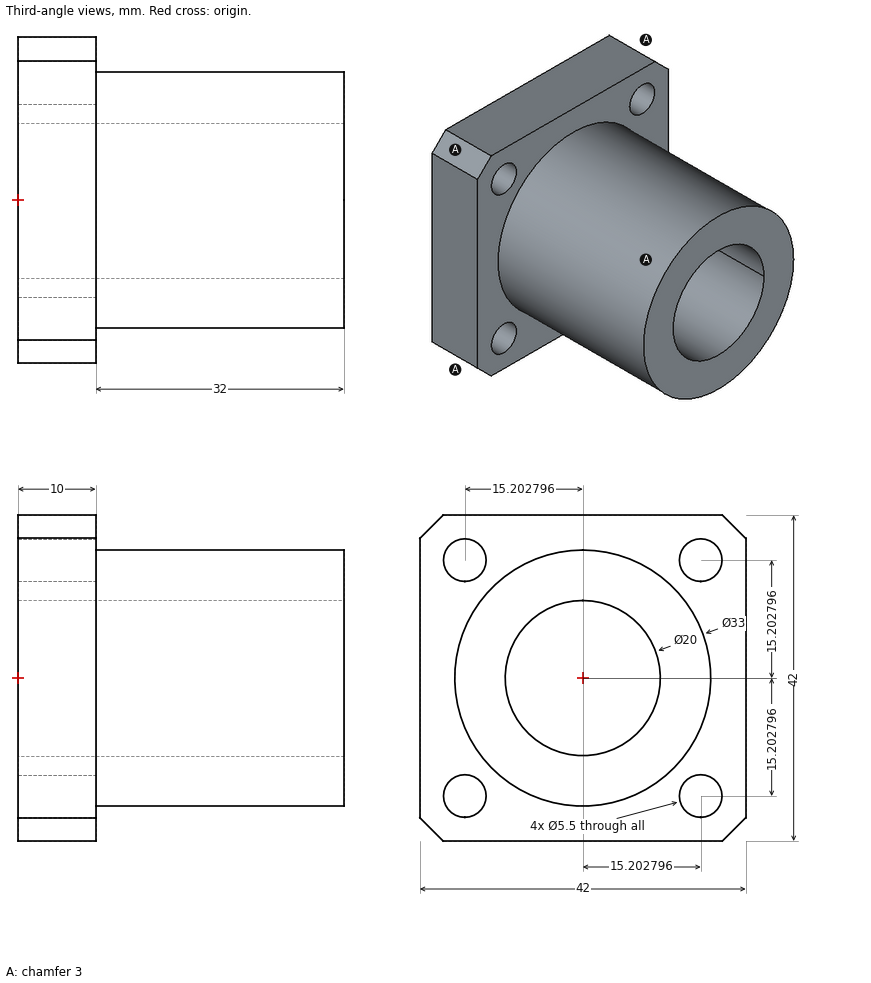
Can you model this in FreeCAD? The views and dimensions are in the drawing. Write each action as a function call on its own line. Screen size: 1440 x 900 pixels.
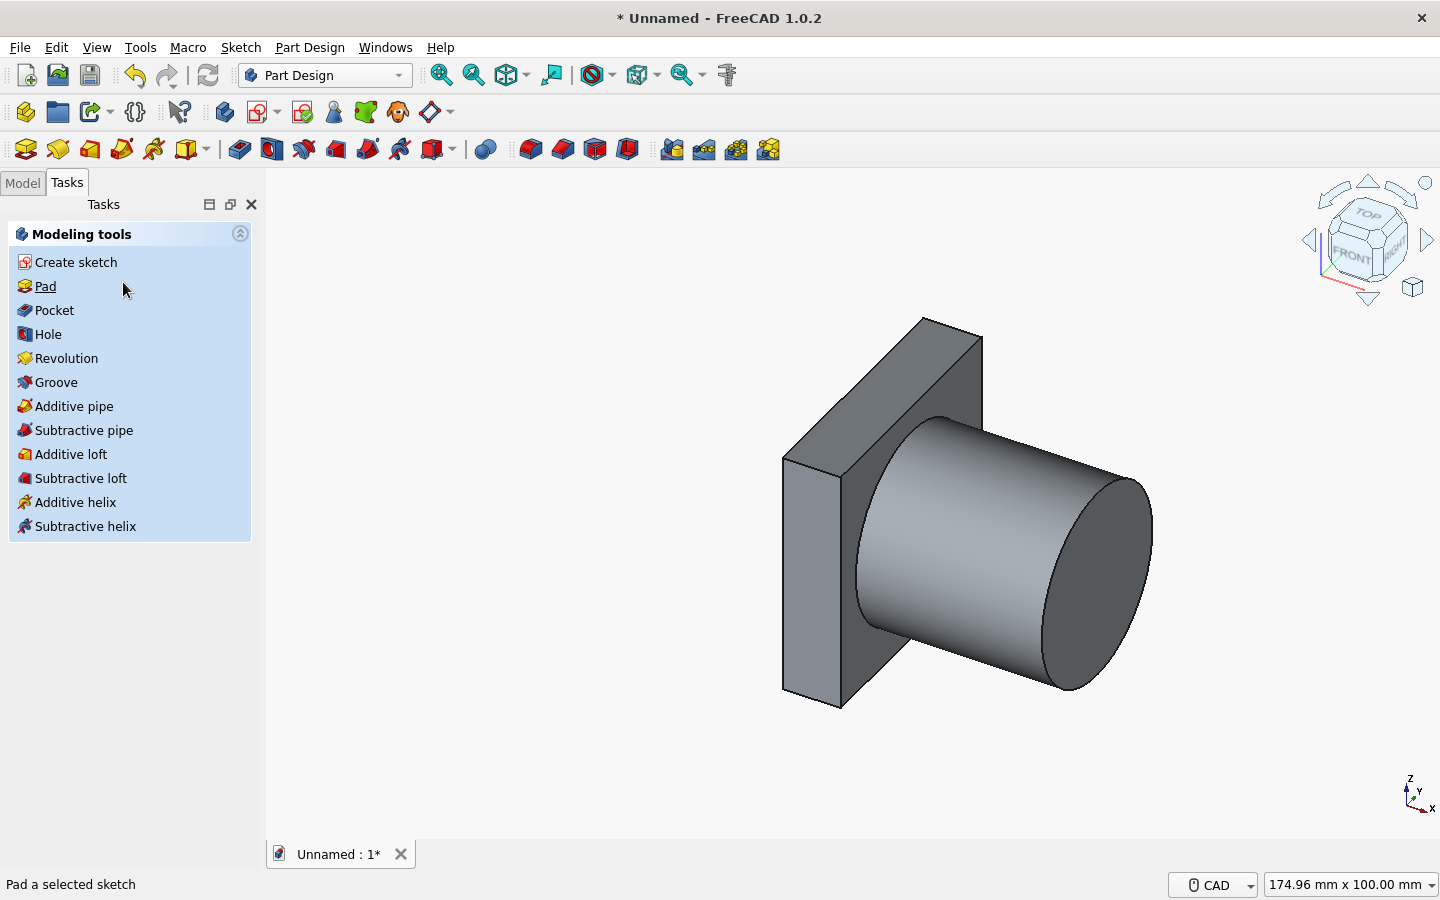
click(272, 150)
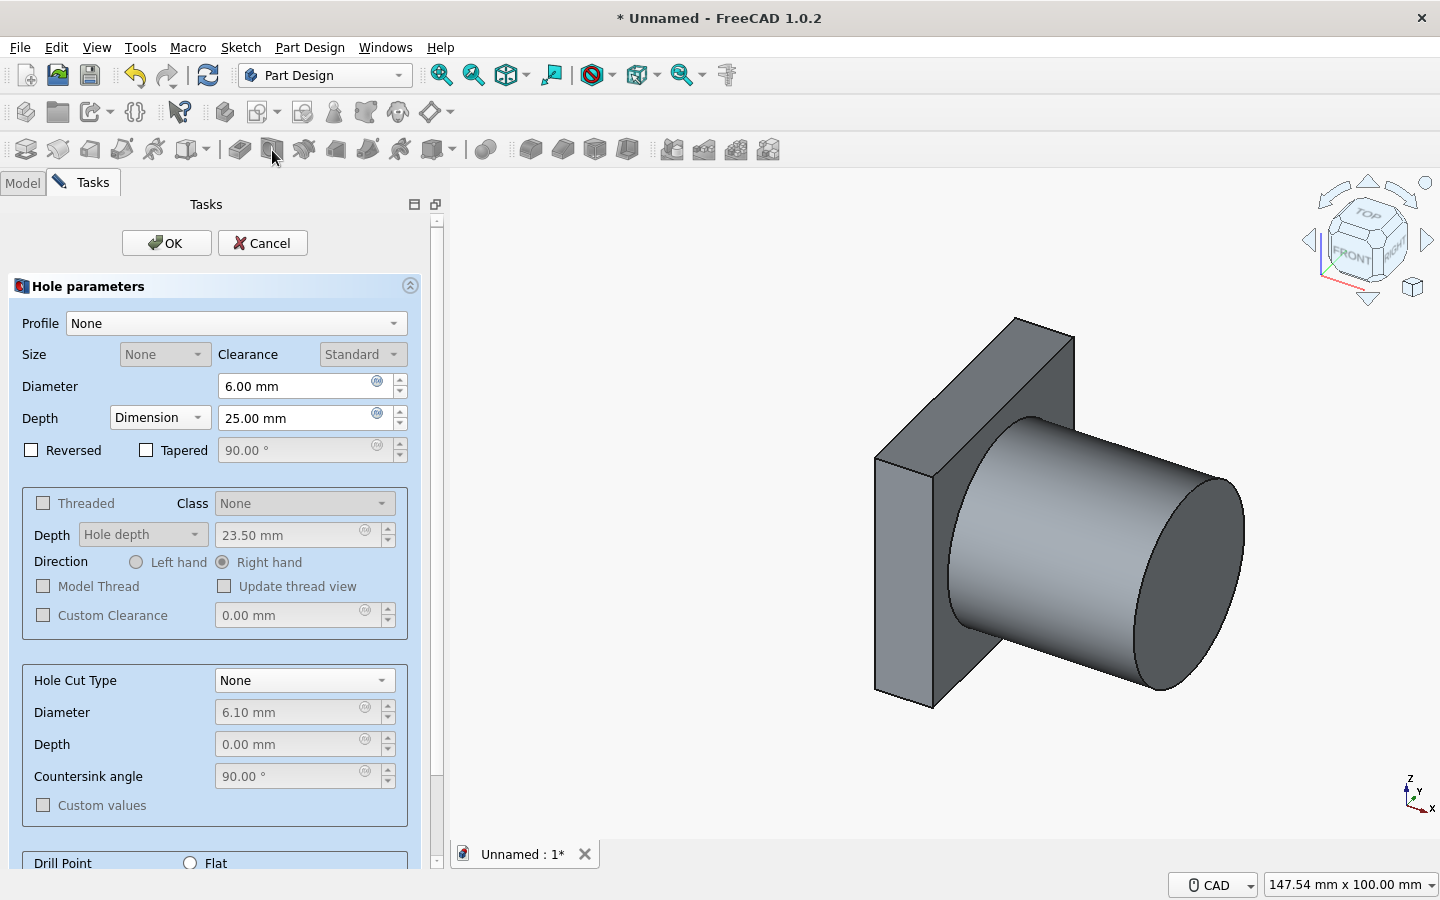
triple_click(305, 386)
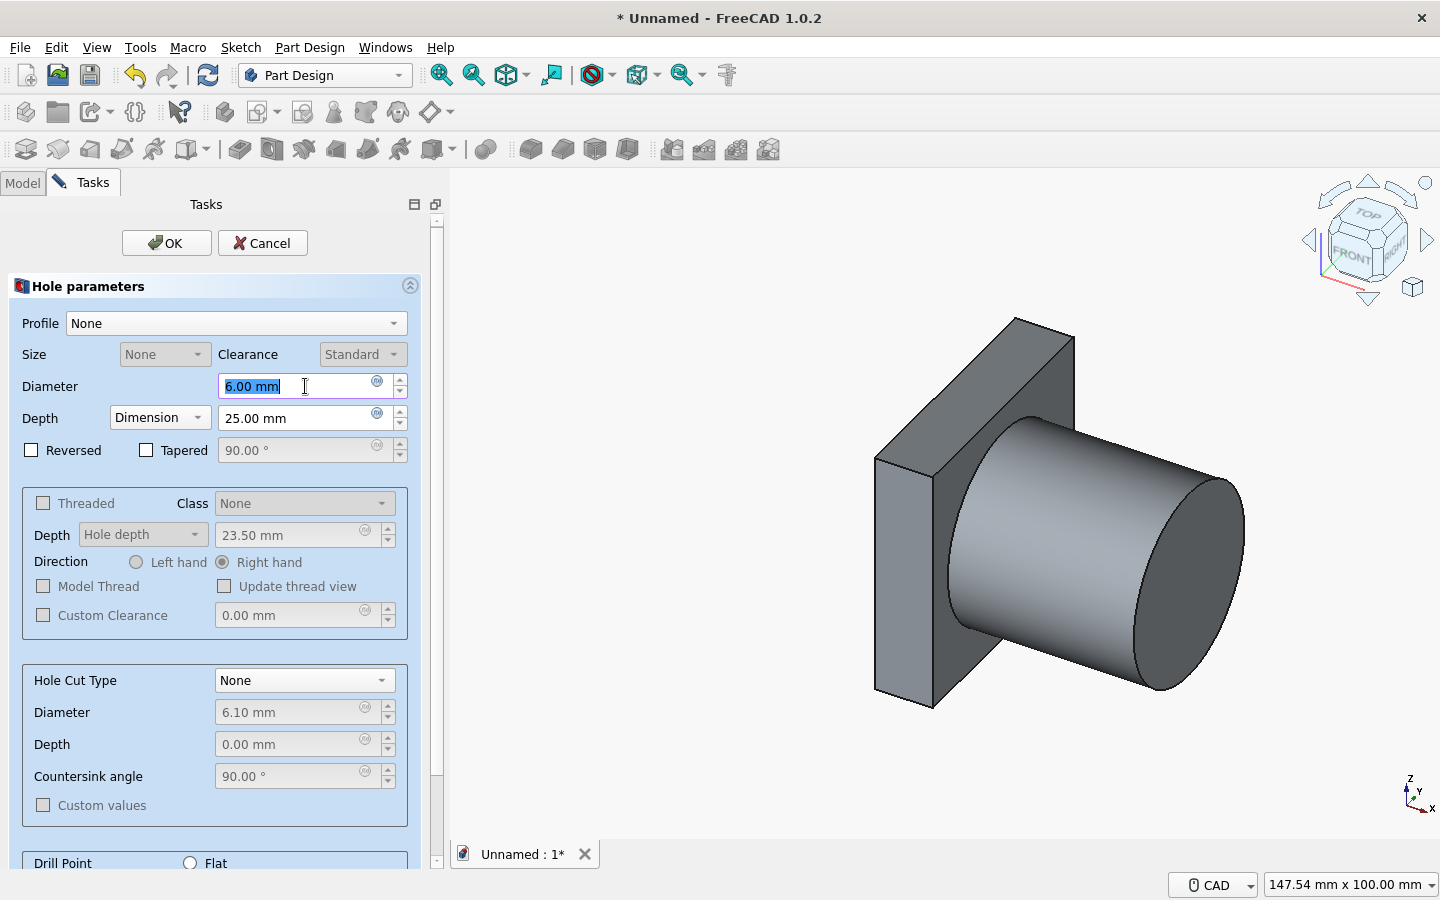
text(5.5)
key(Tab)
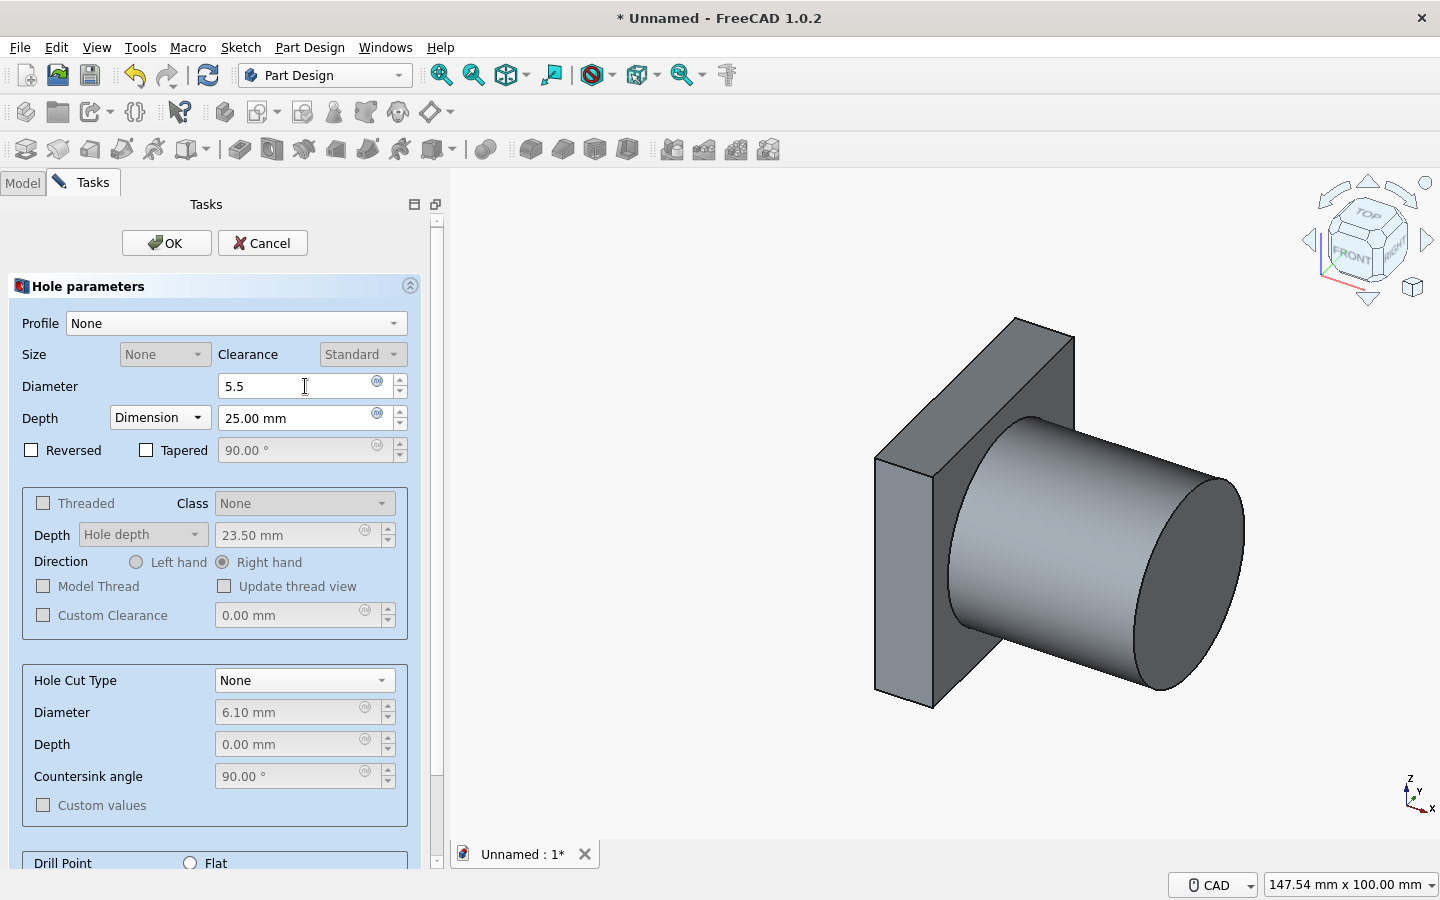
click(161, 418)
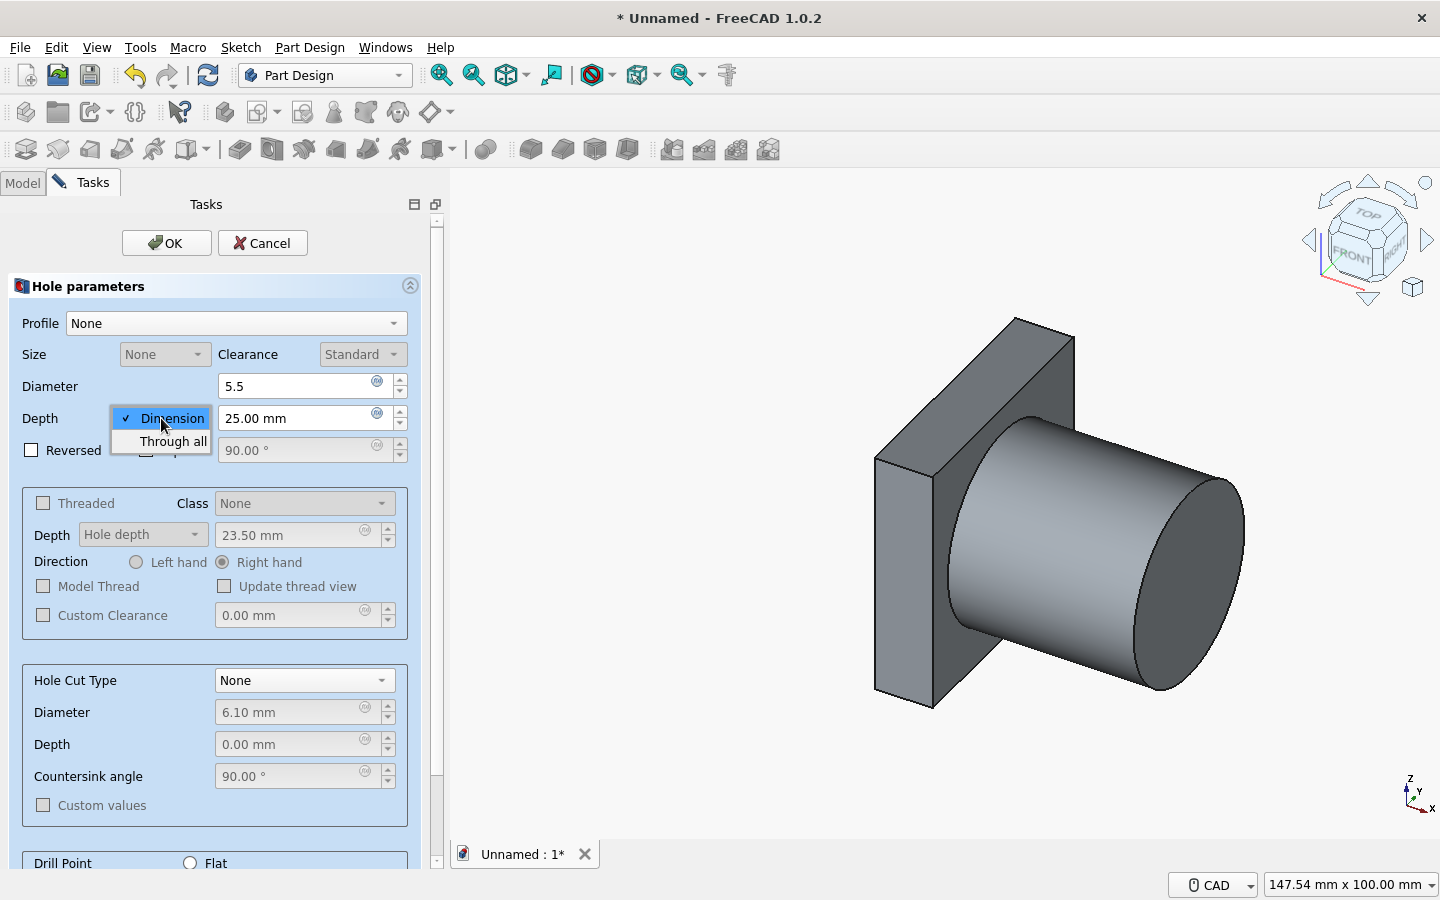
click(160, 442)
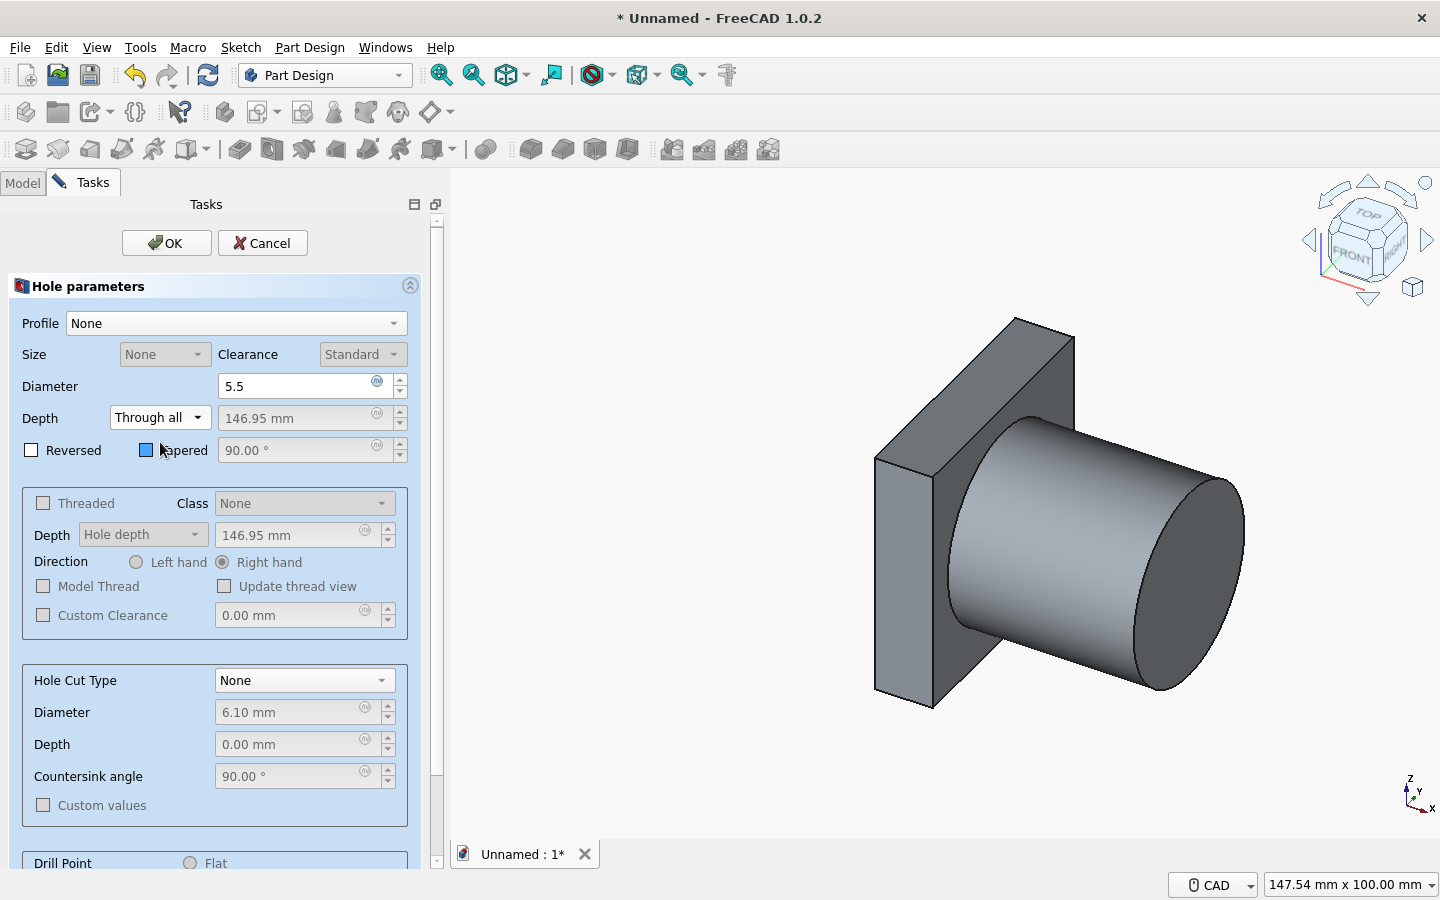
click(30, 450)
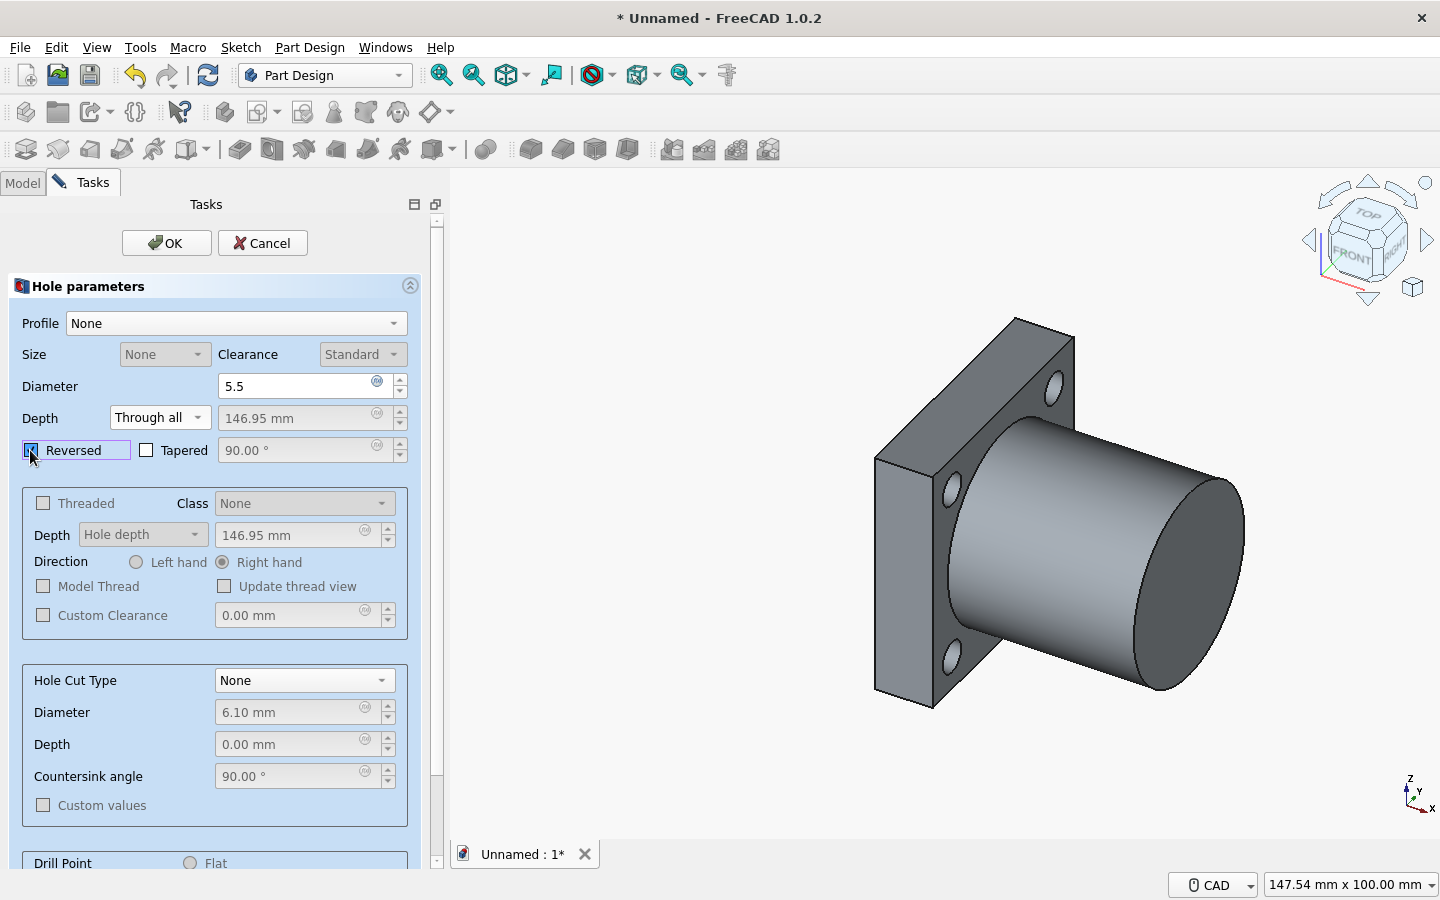
click(167, 243)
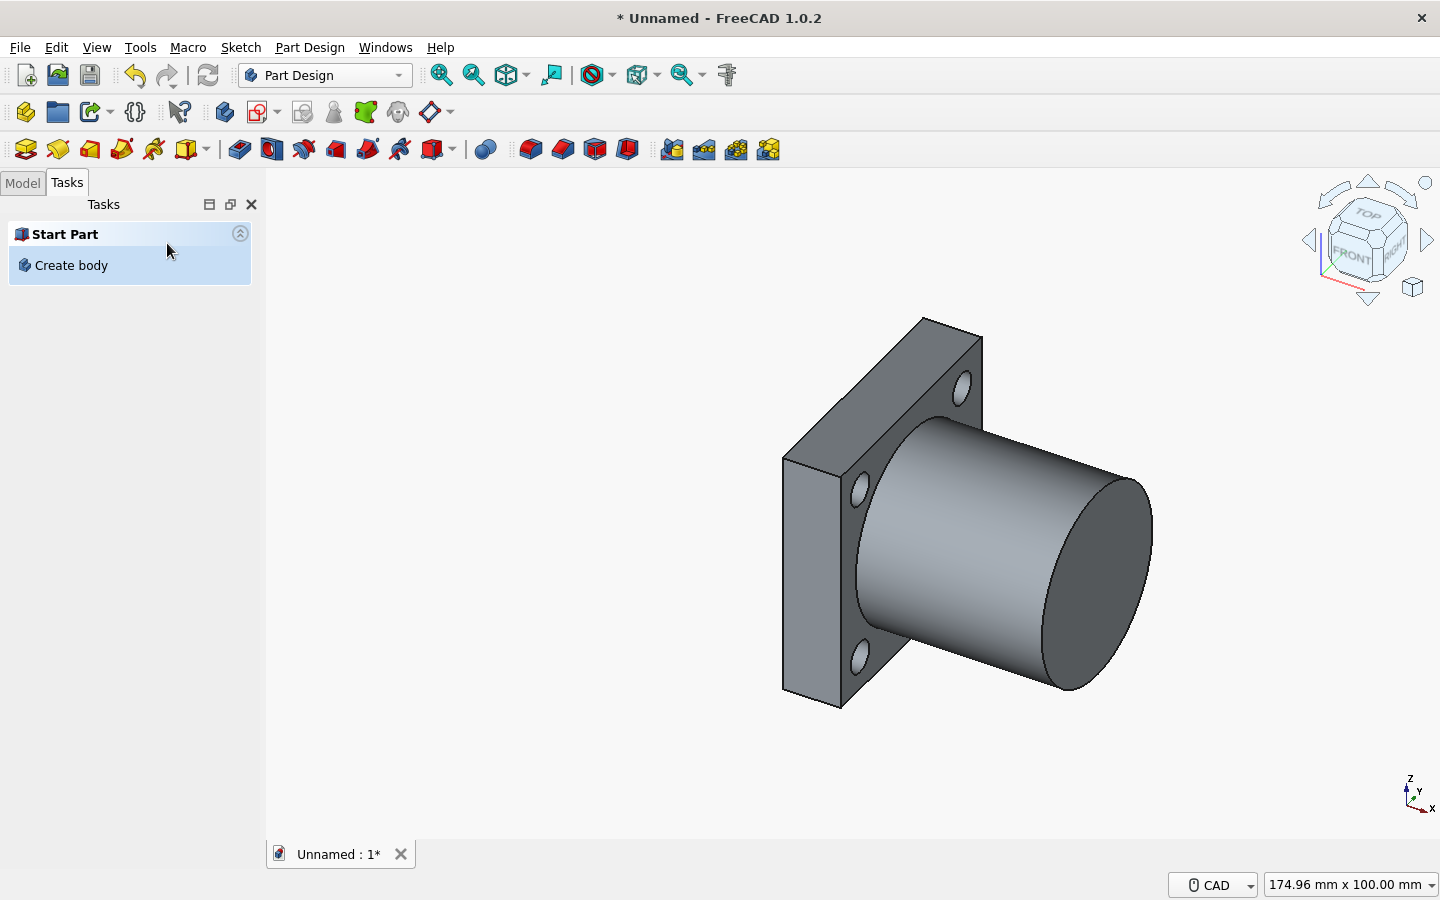
key(6)